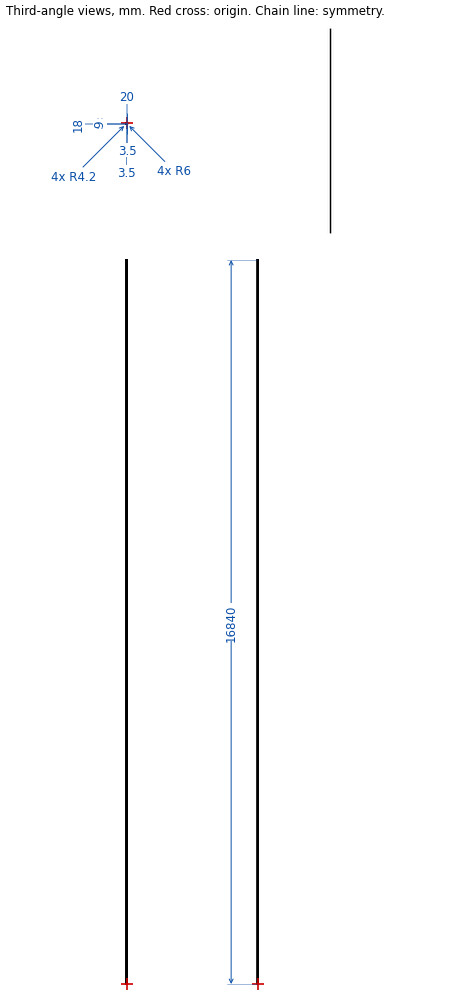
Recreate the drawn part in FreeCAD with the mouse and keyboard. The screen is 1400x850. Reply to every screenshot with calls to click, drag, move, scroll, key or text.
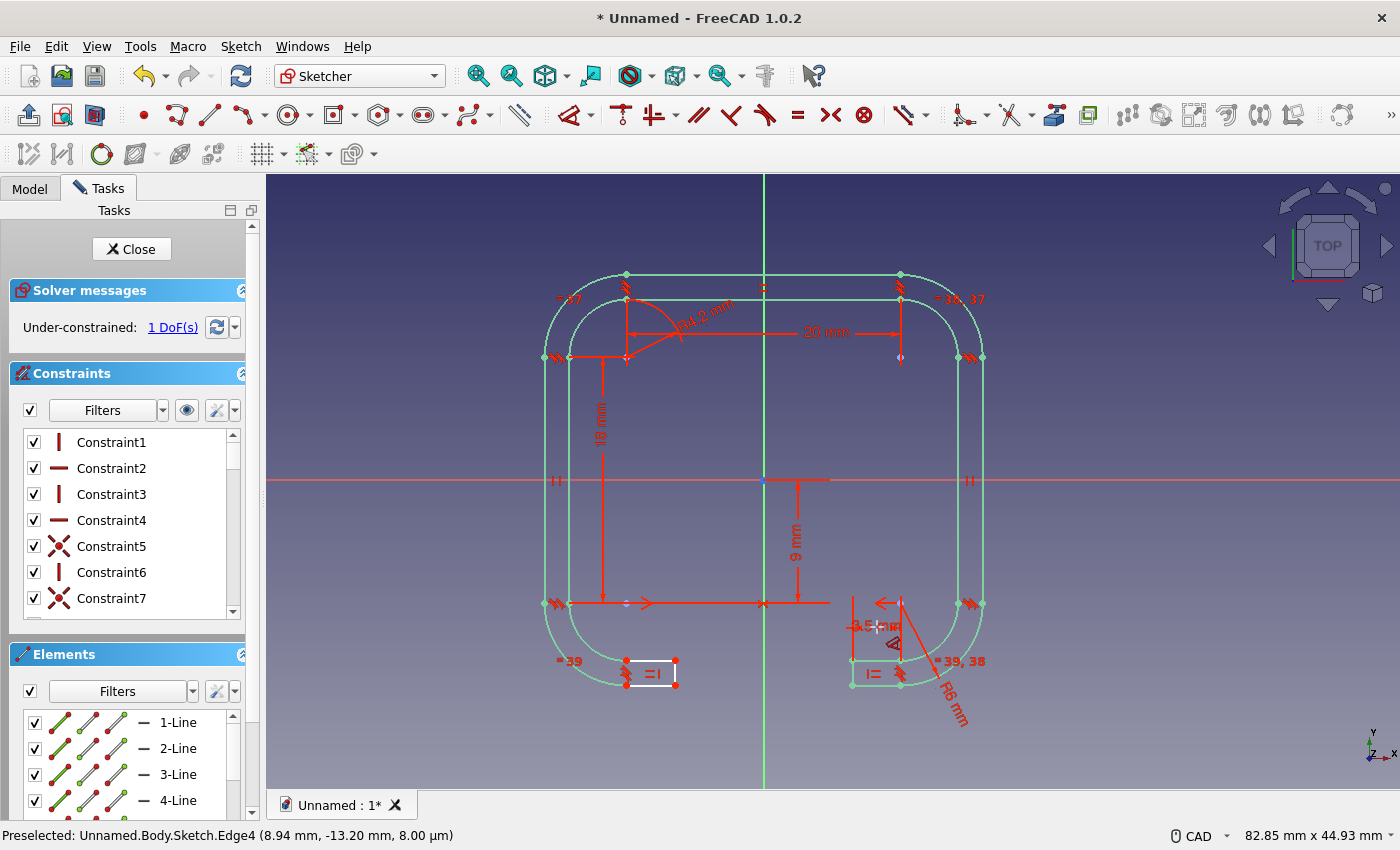
click(641, 686)
click(651, 720)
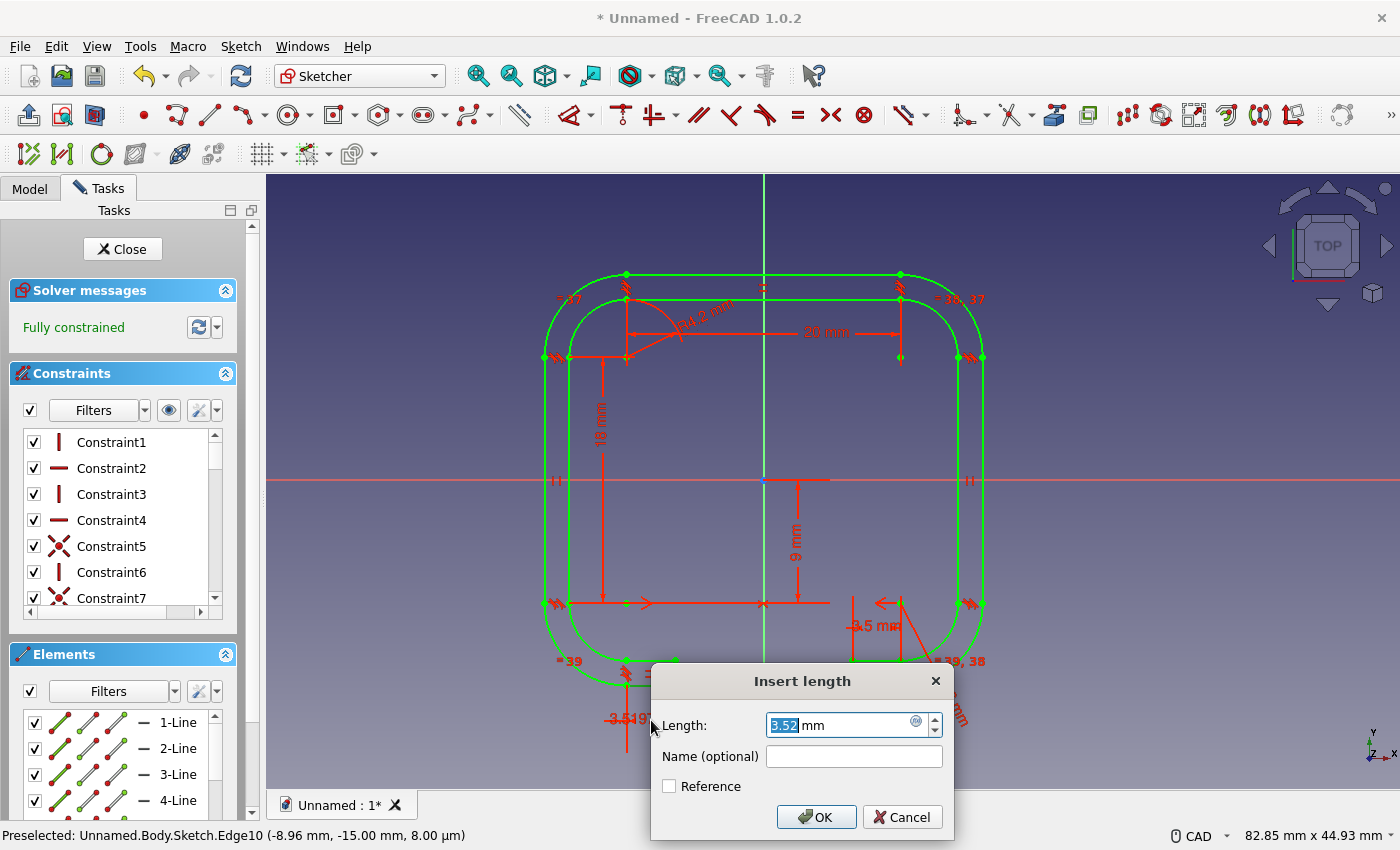
text(3.5)
key(Return)
key(Escape)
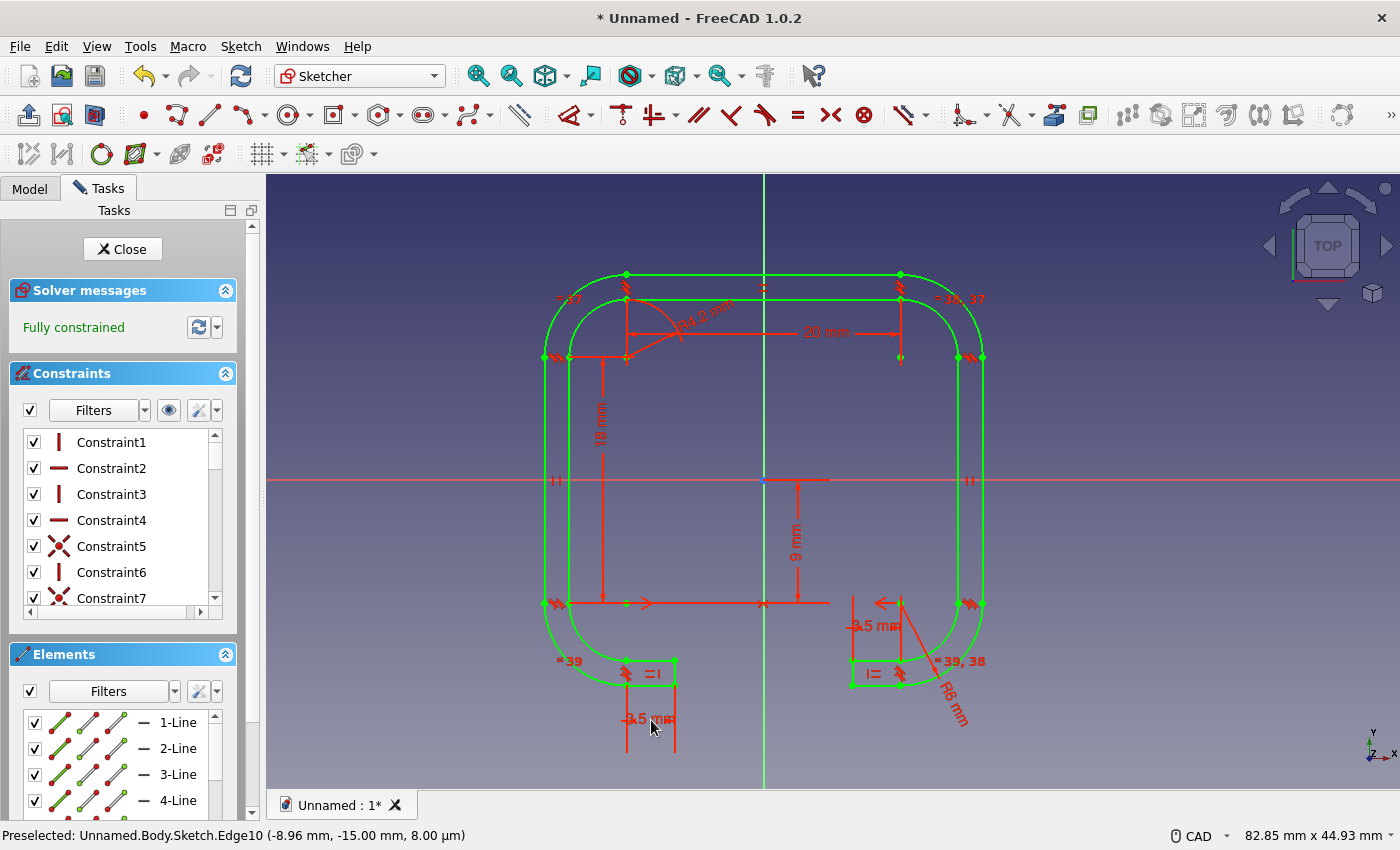
click(123, 249)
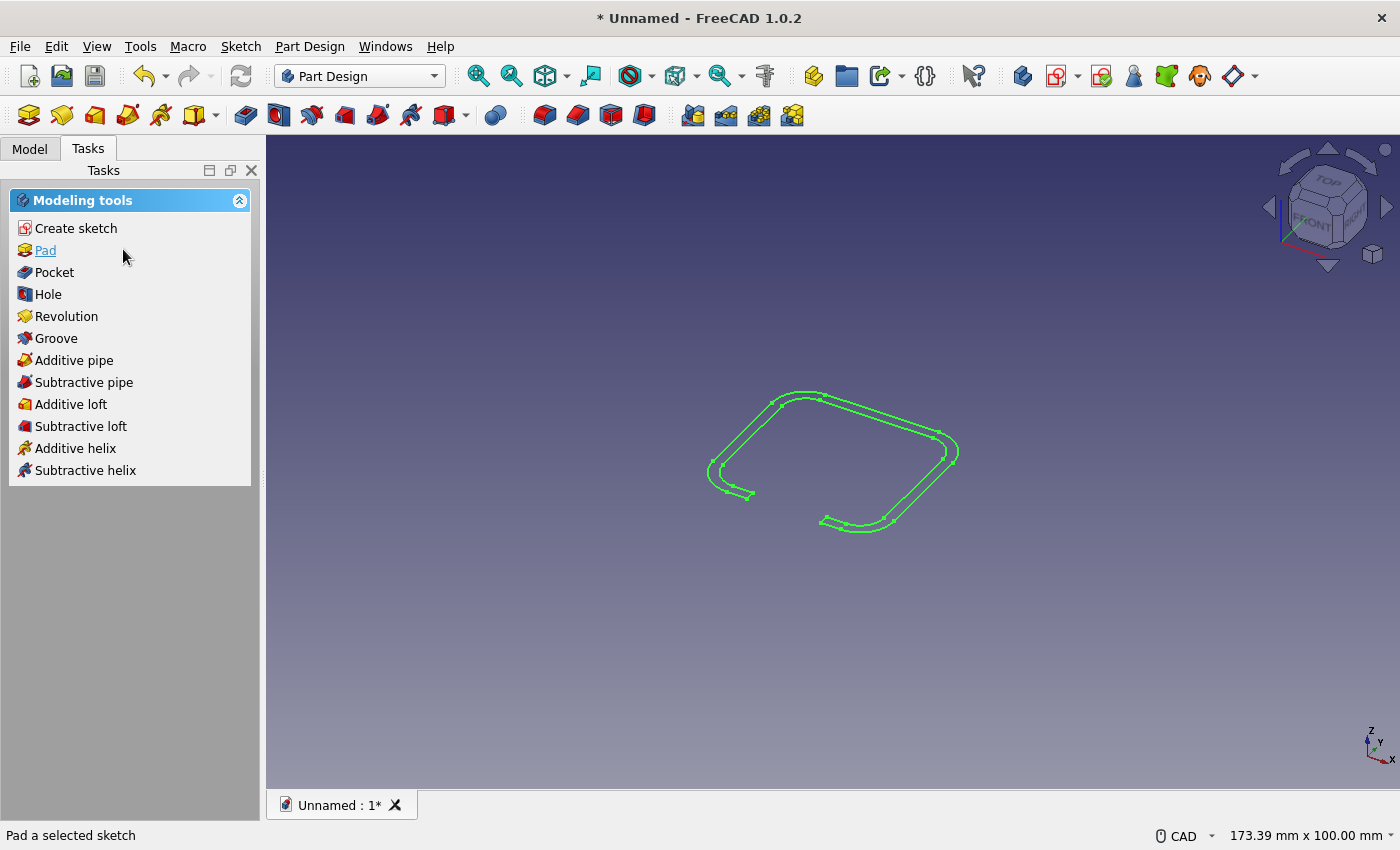
click(29, 116)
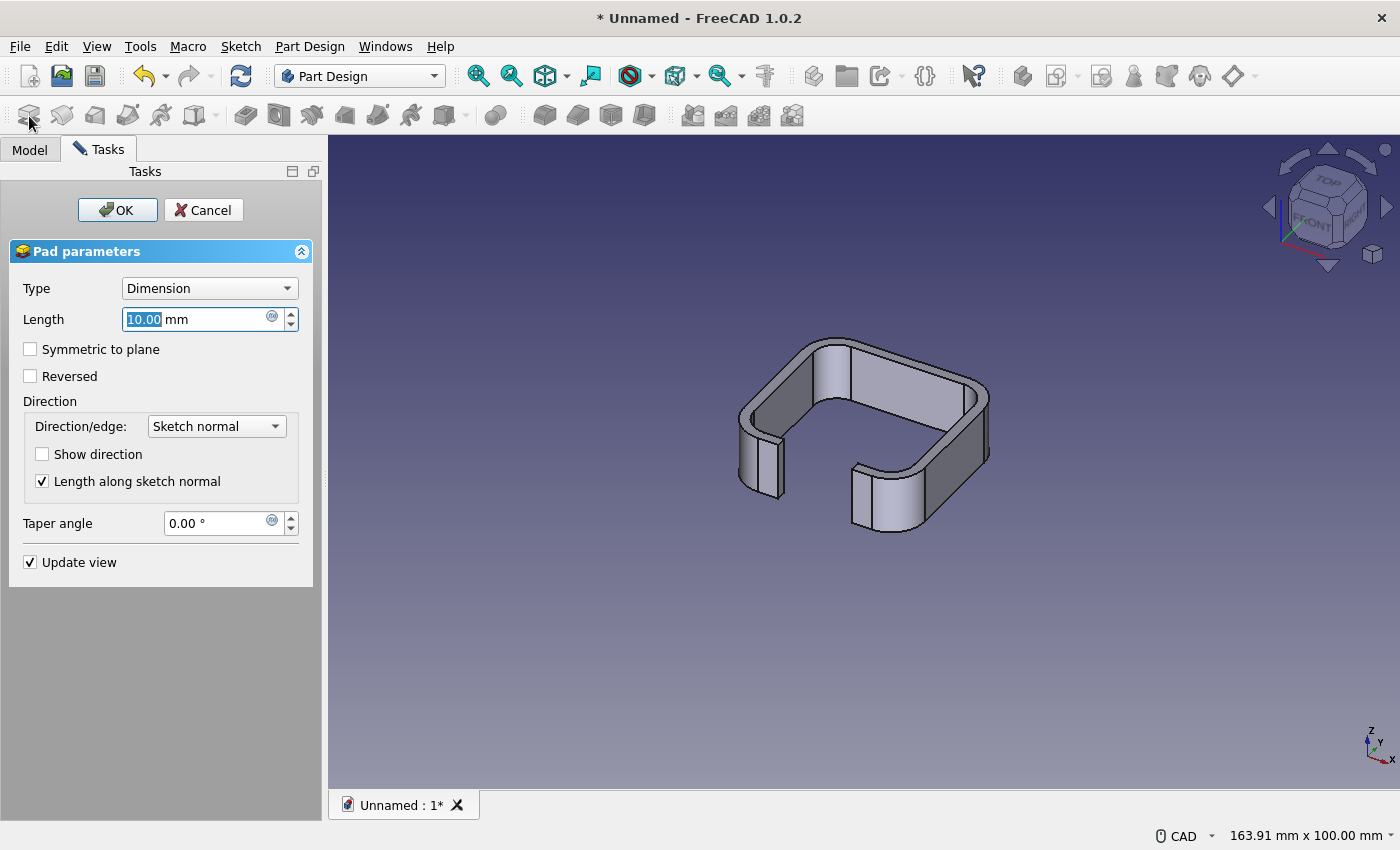
text(16840)
key(Tab)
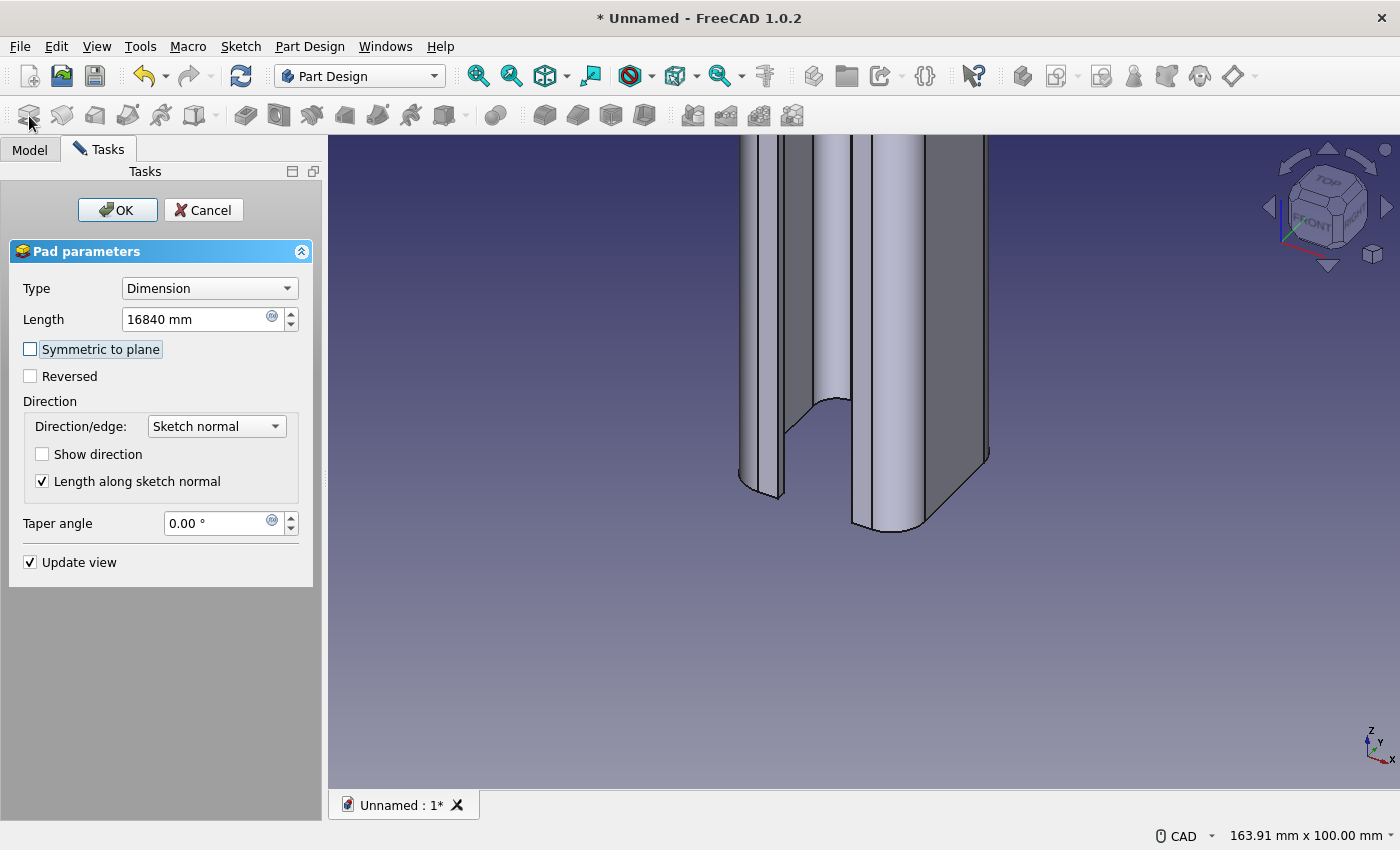
click(118, 210)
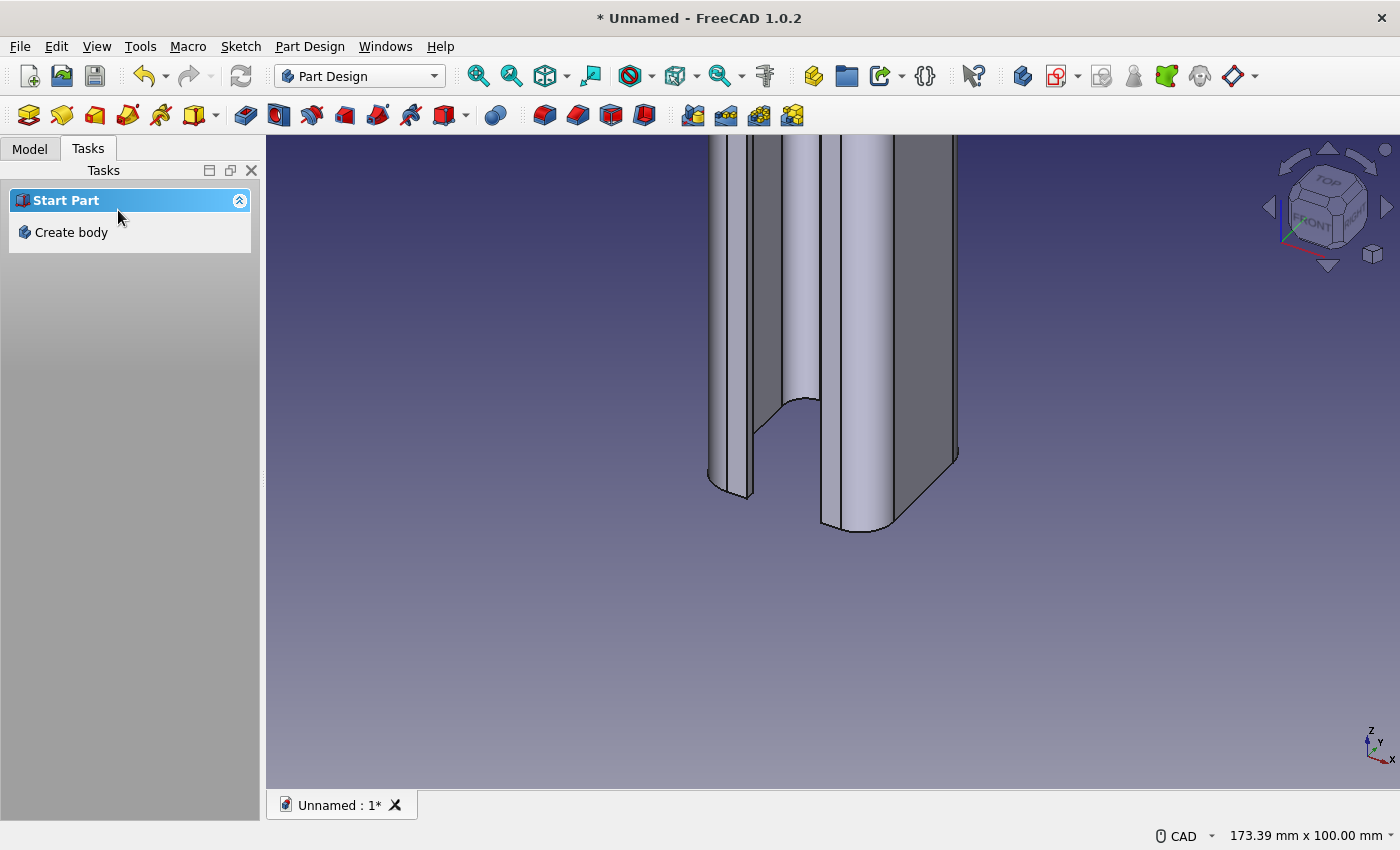
key(0)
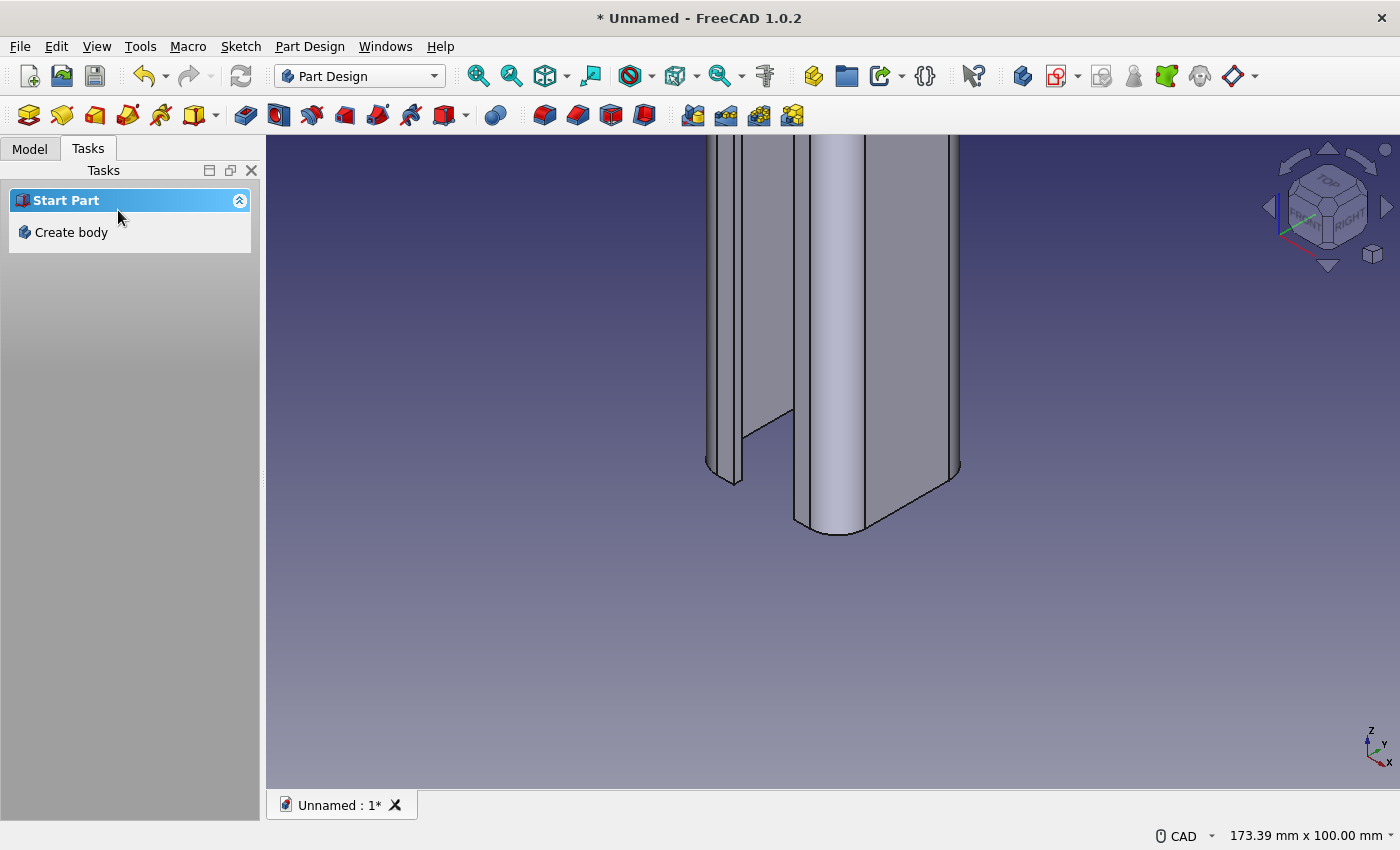
click(479, 76)